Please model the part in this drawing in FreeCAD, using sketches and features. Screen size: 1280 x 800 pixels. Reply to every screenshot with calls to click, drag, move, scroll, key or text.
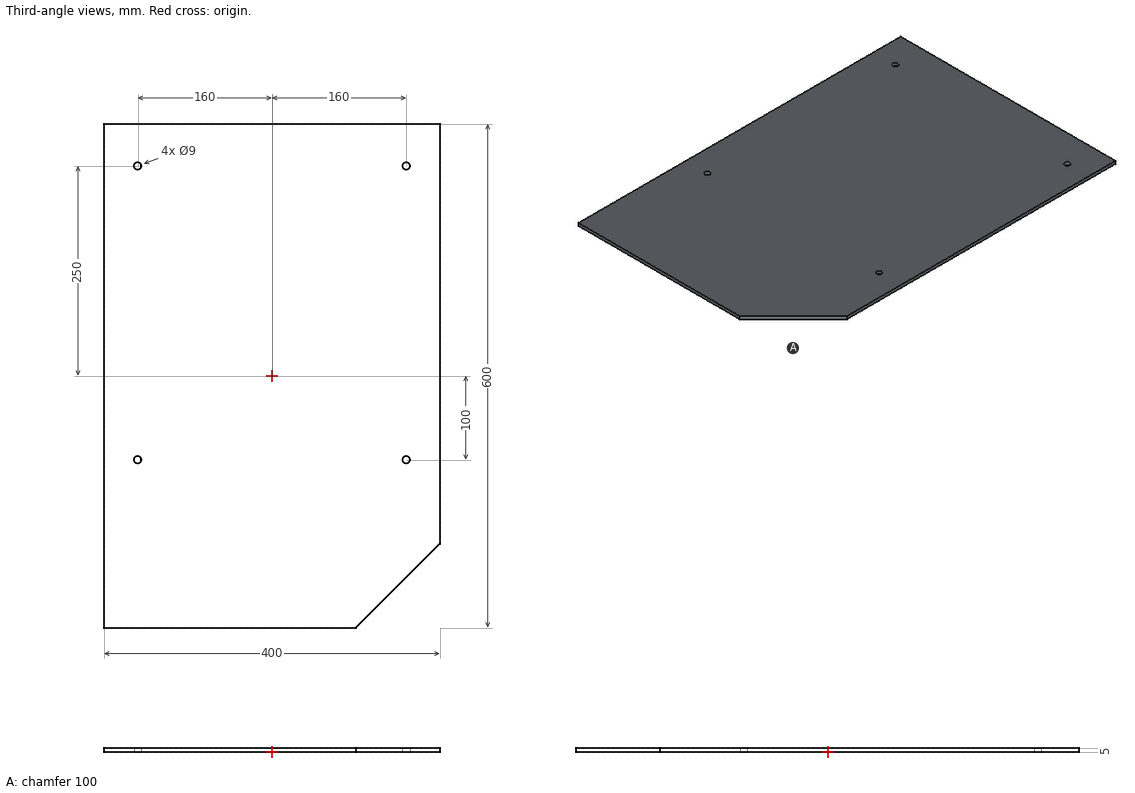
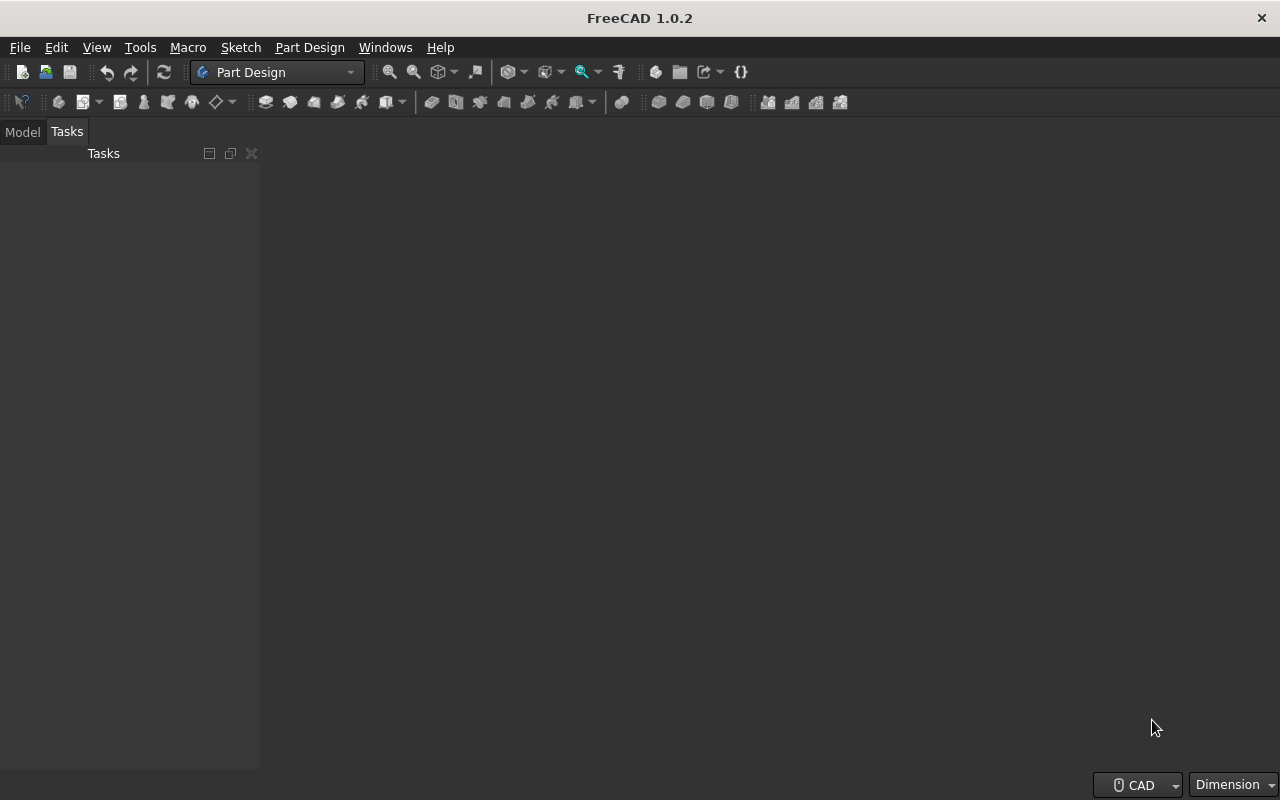
click(22, 72)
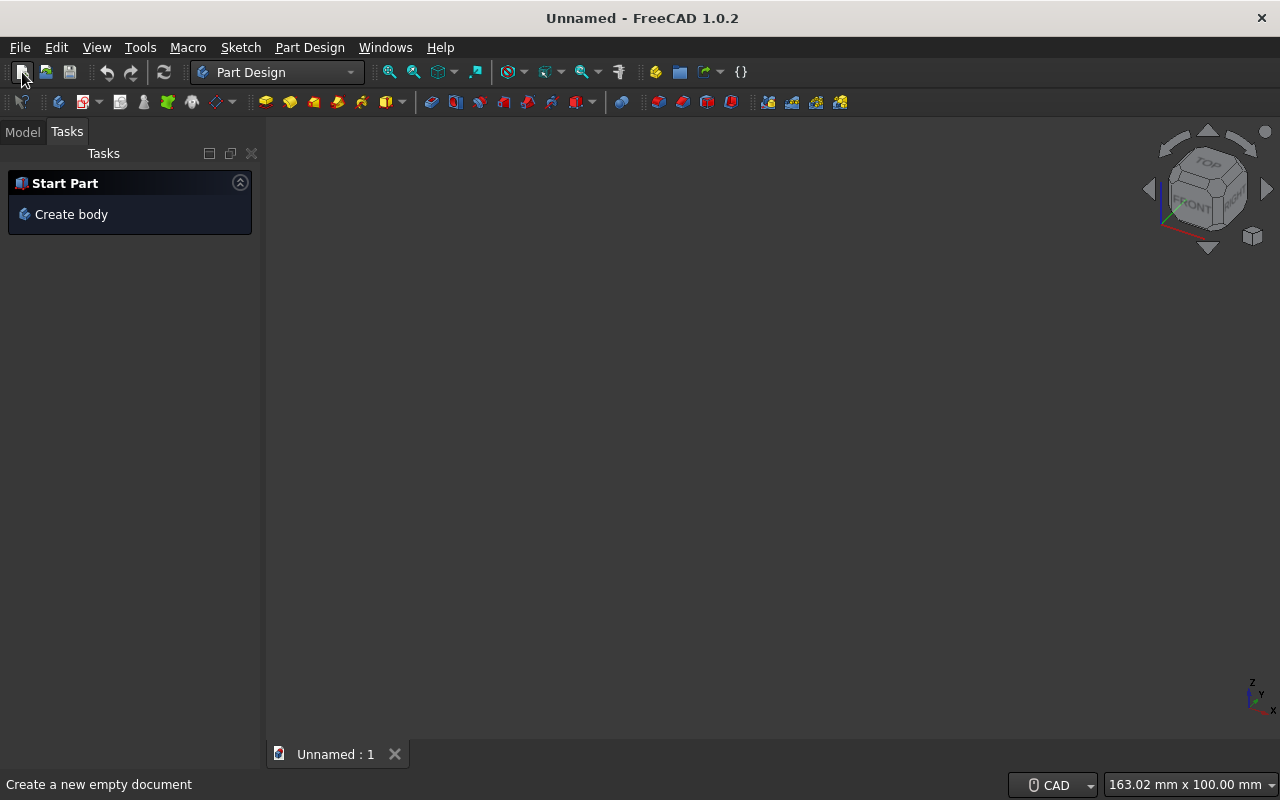
click(84, 102)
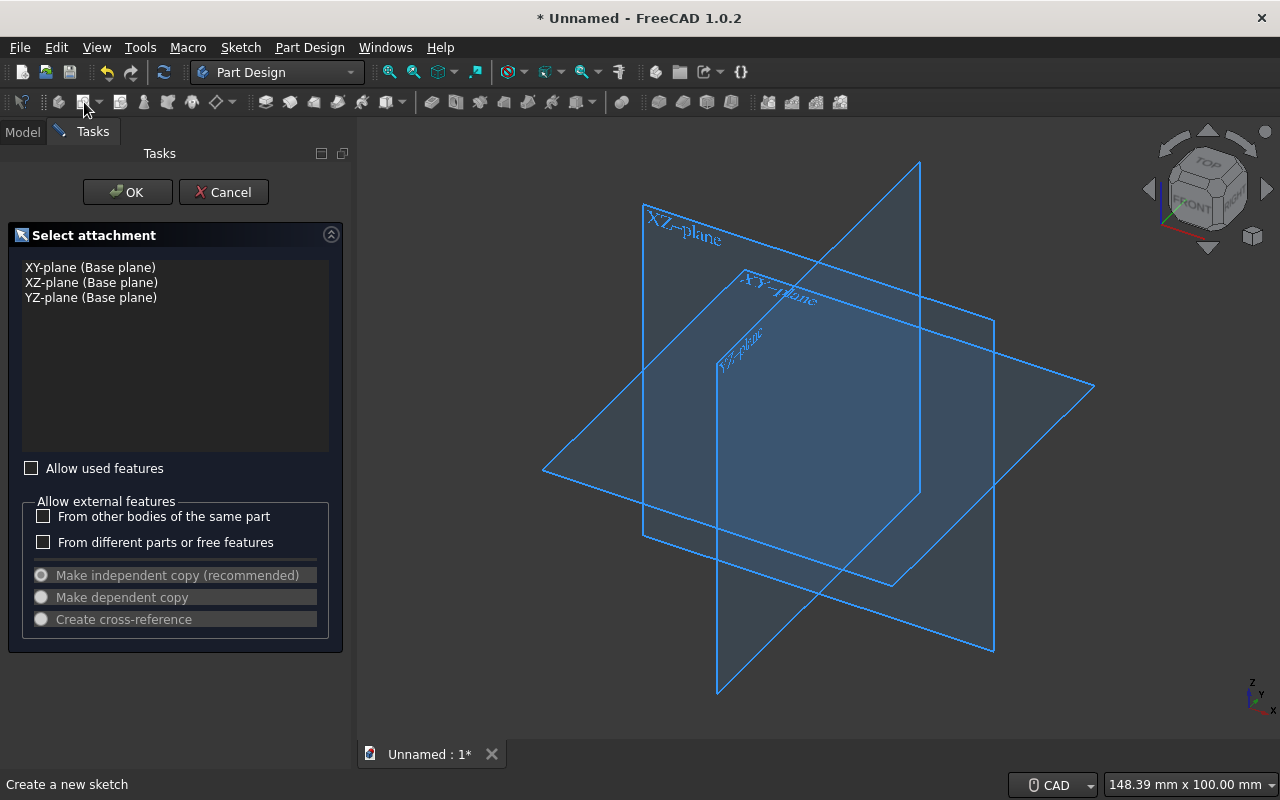
click(82, 268)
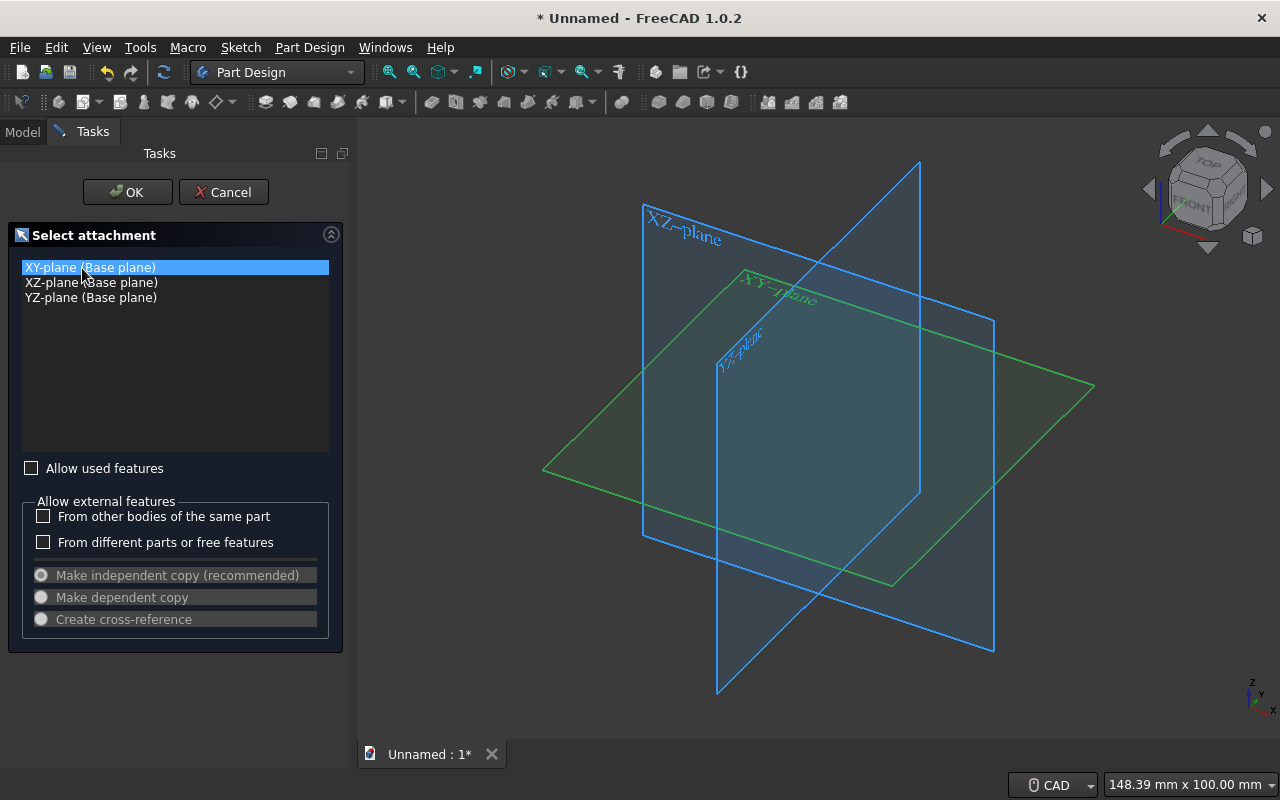
click(128, 192)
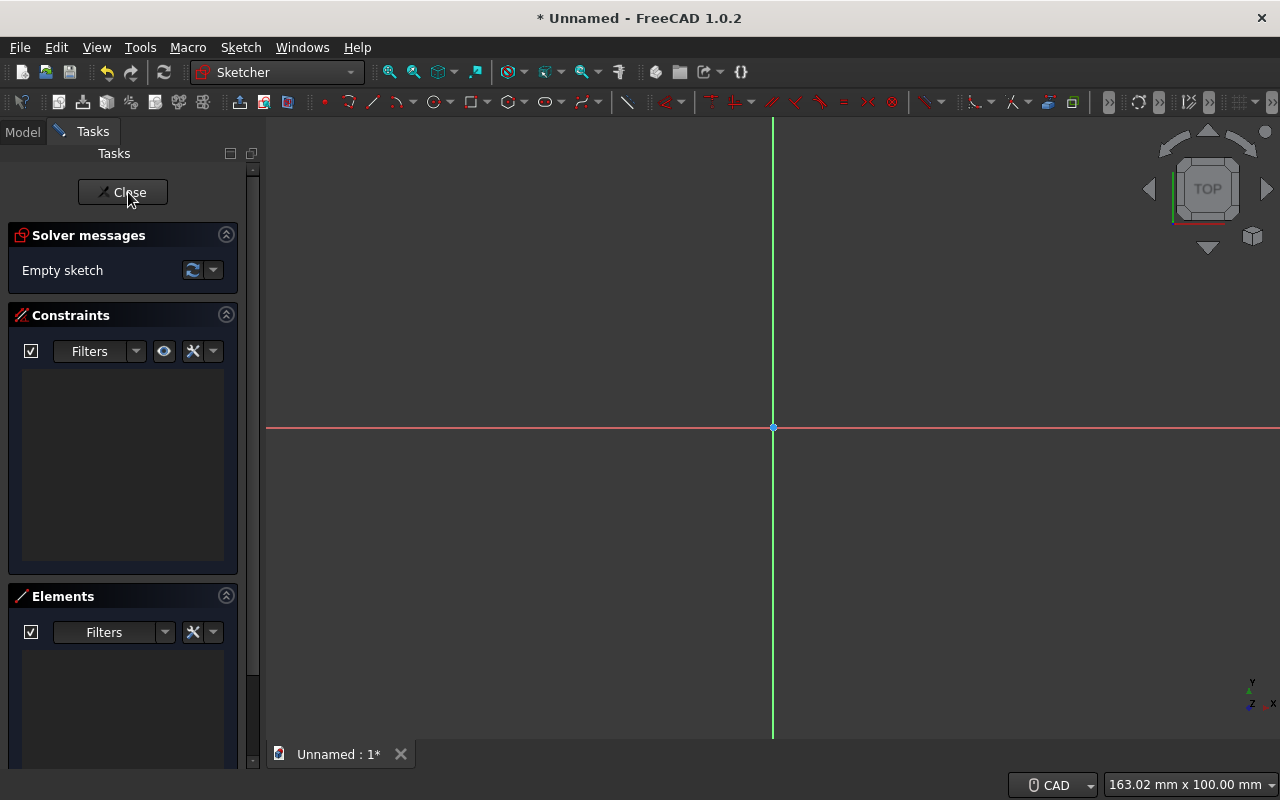
scroll(696, 428, down, 11)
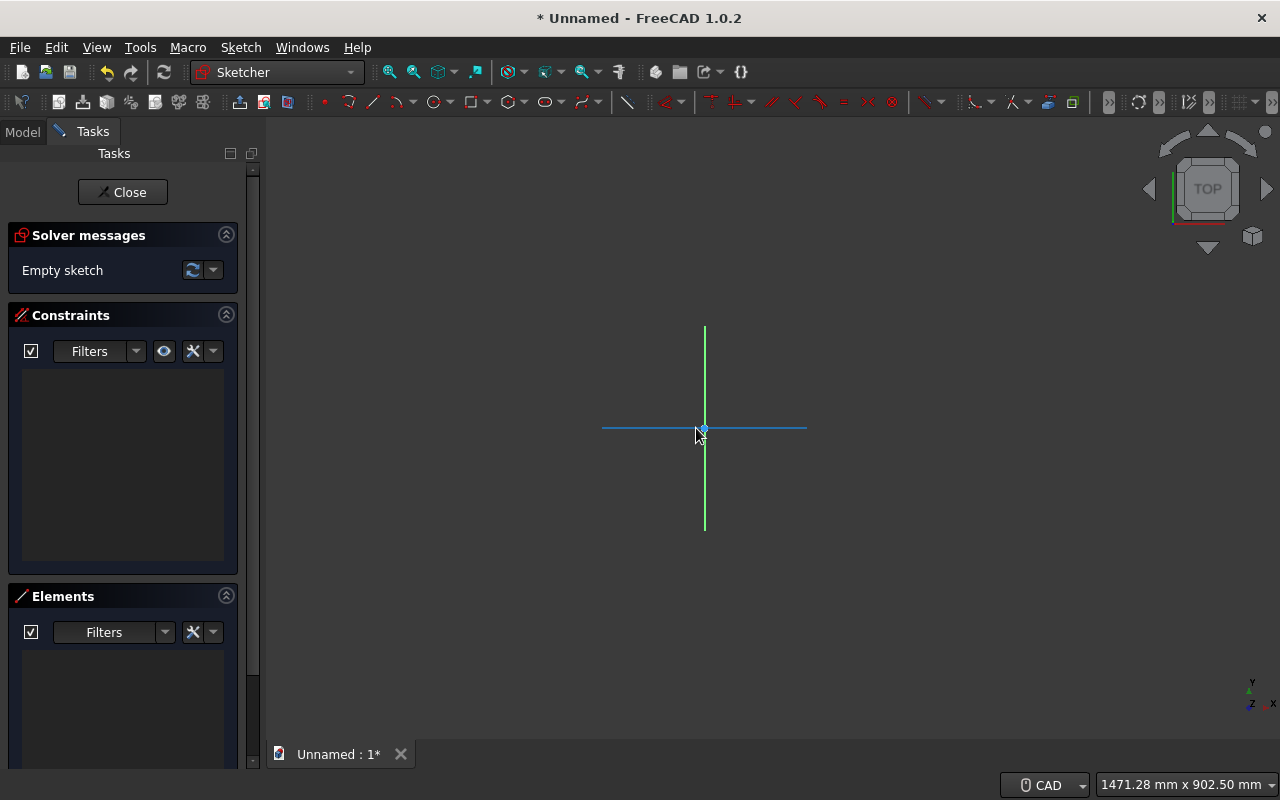
click(490, 102)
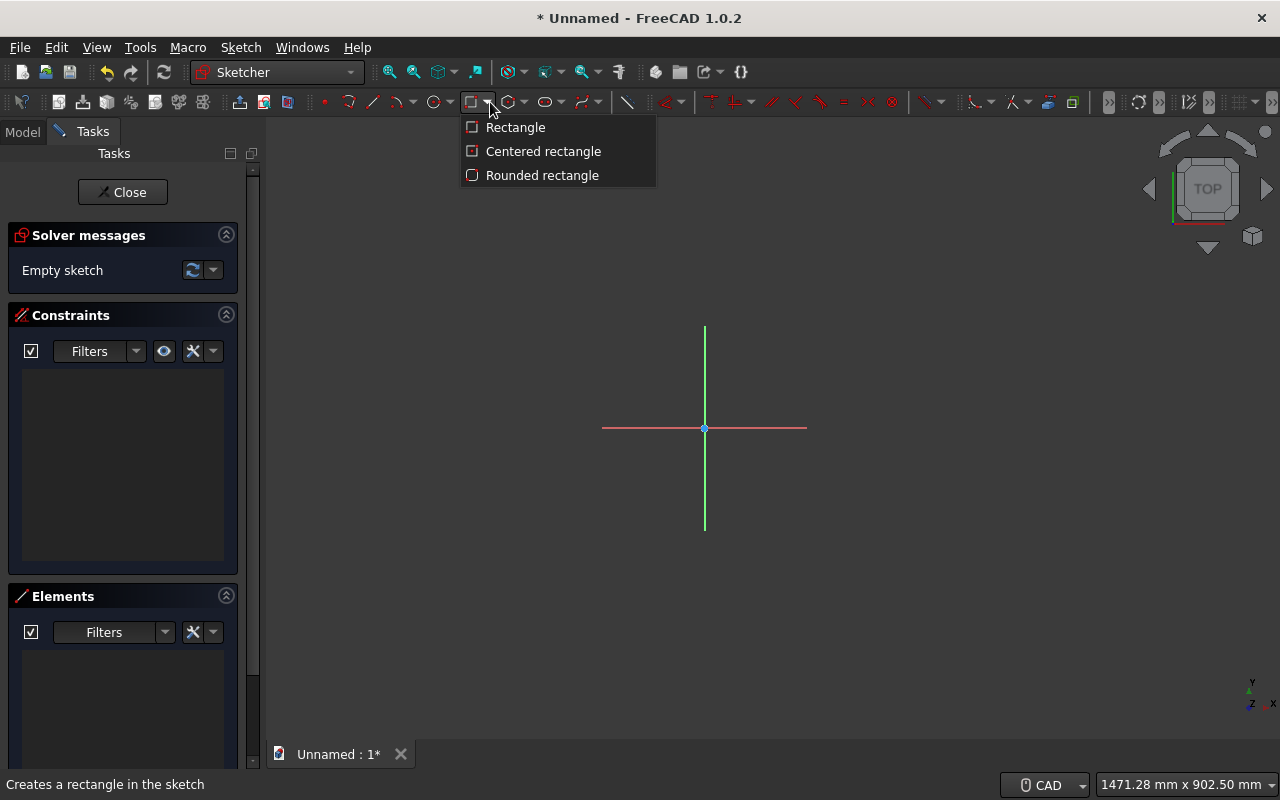
click(558, 151)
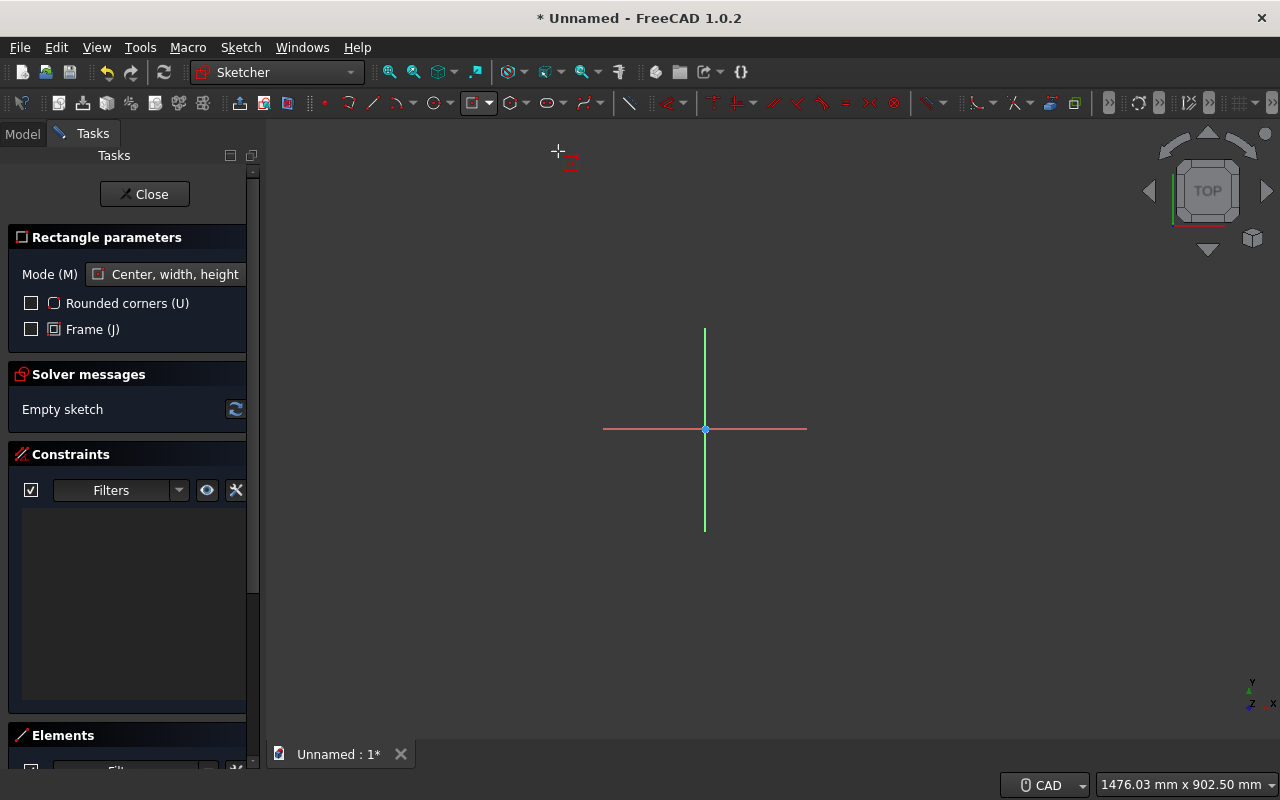
click(705, 429)
click(843, 223)
key(Escape)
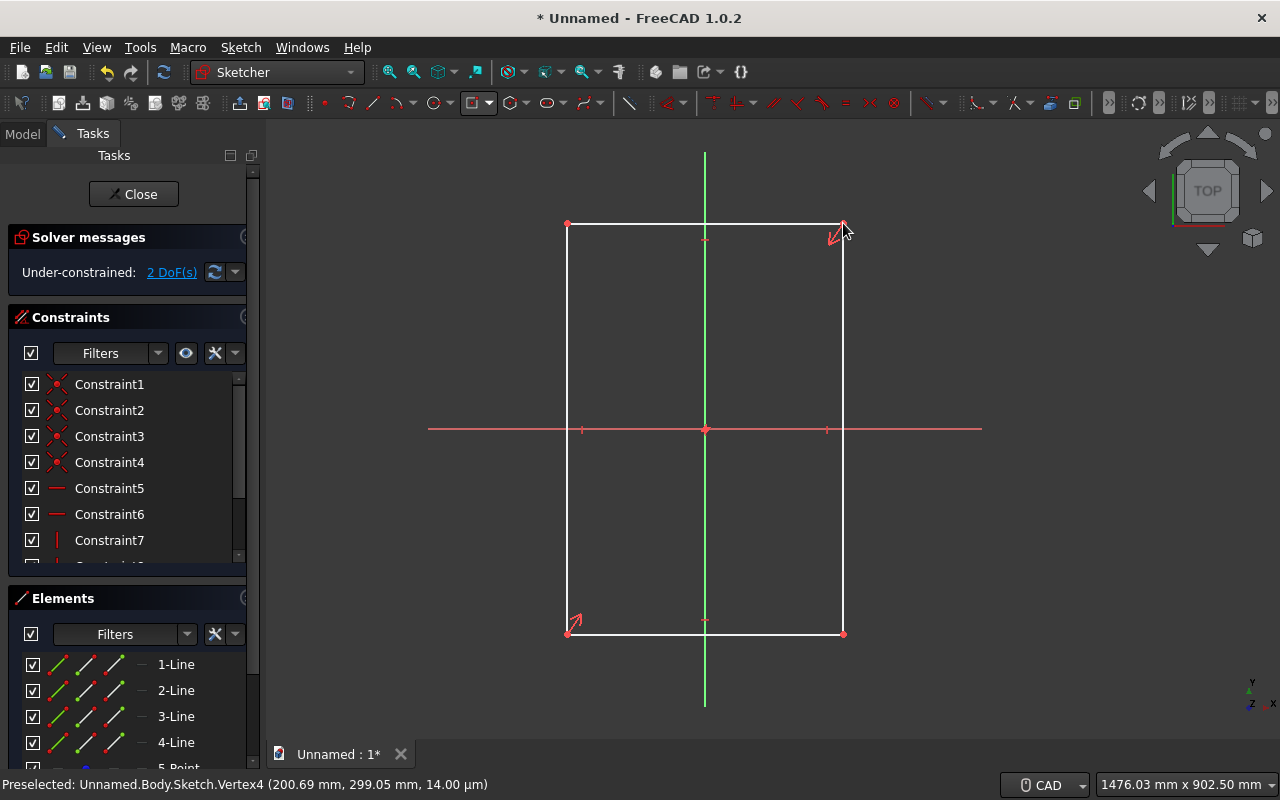
click(668, 104)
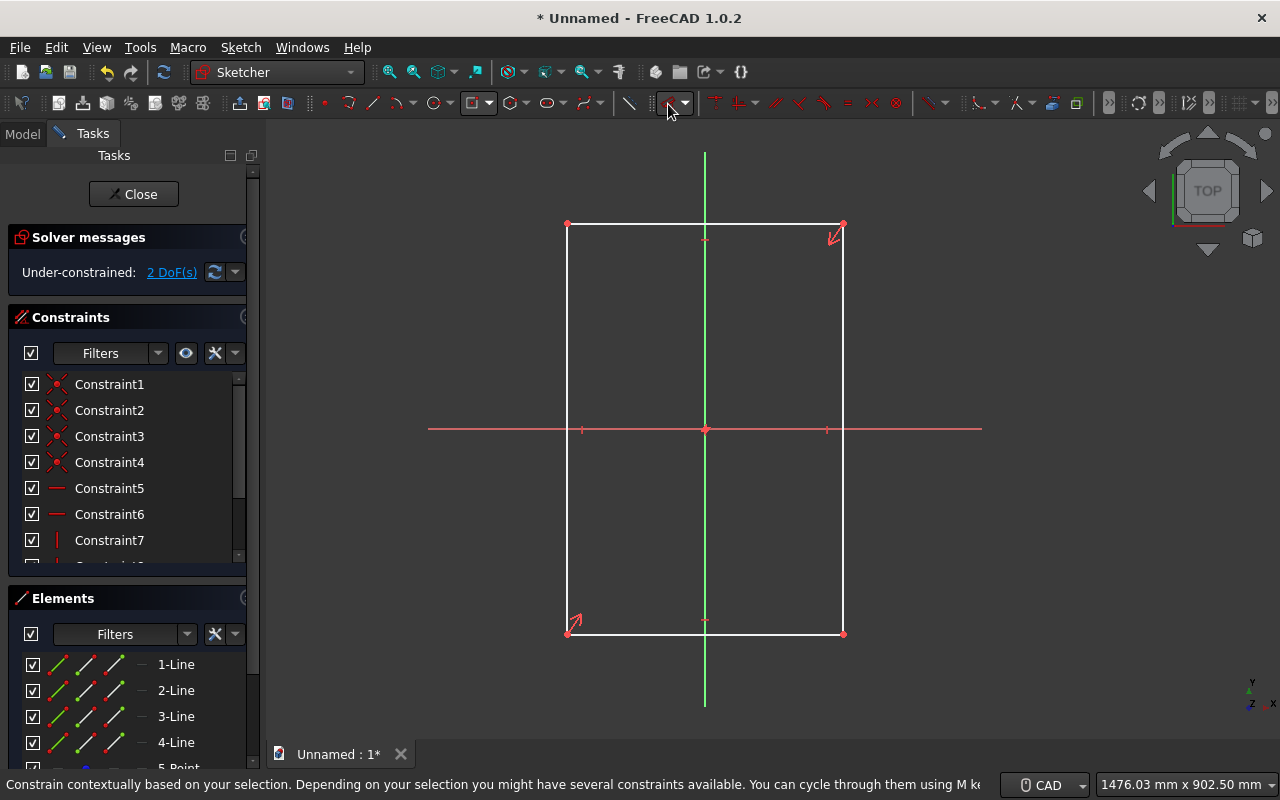
click(650, 635)
click(642, 669)